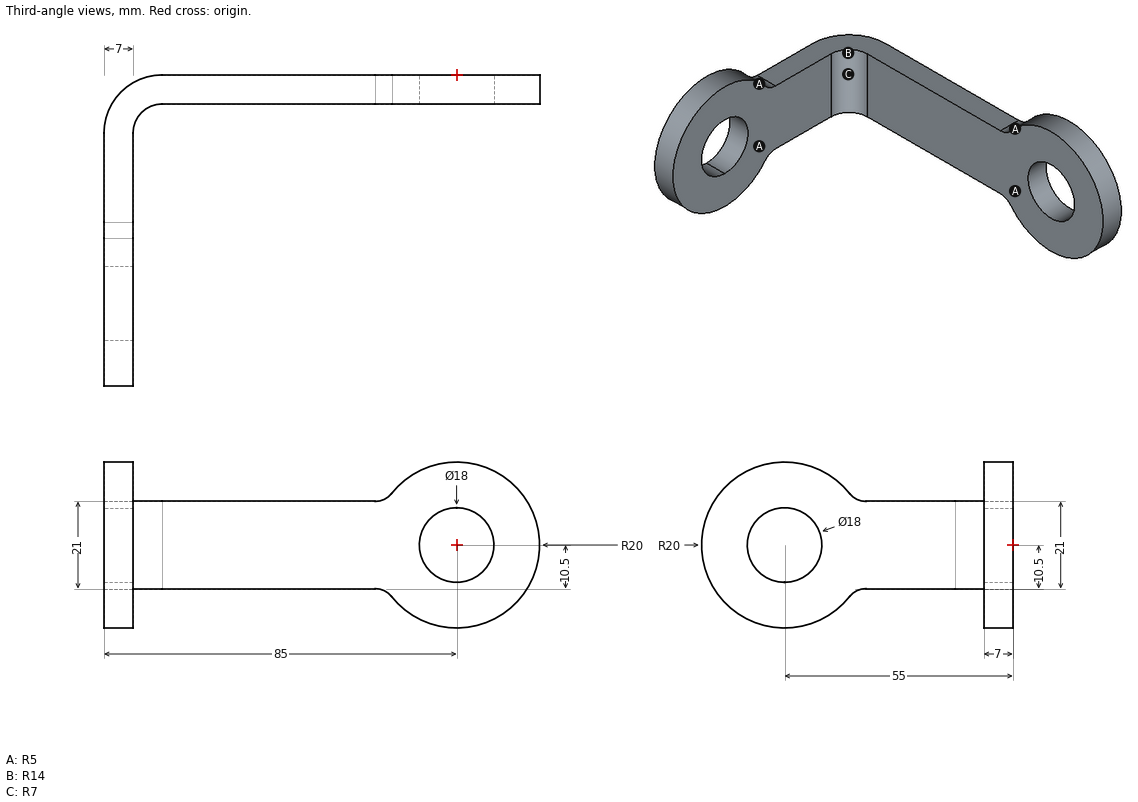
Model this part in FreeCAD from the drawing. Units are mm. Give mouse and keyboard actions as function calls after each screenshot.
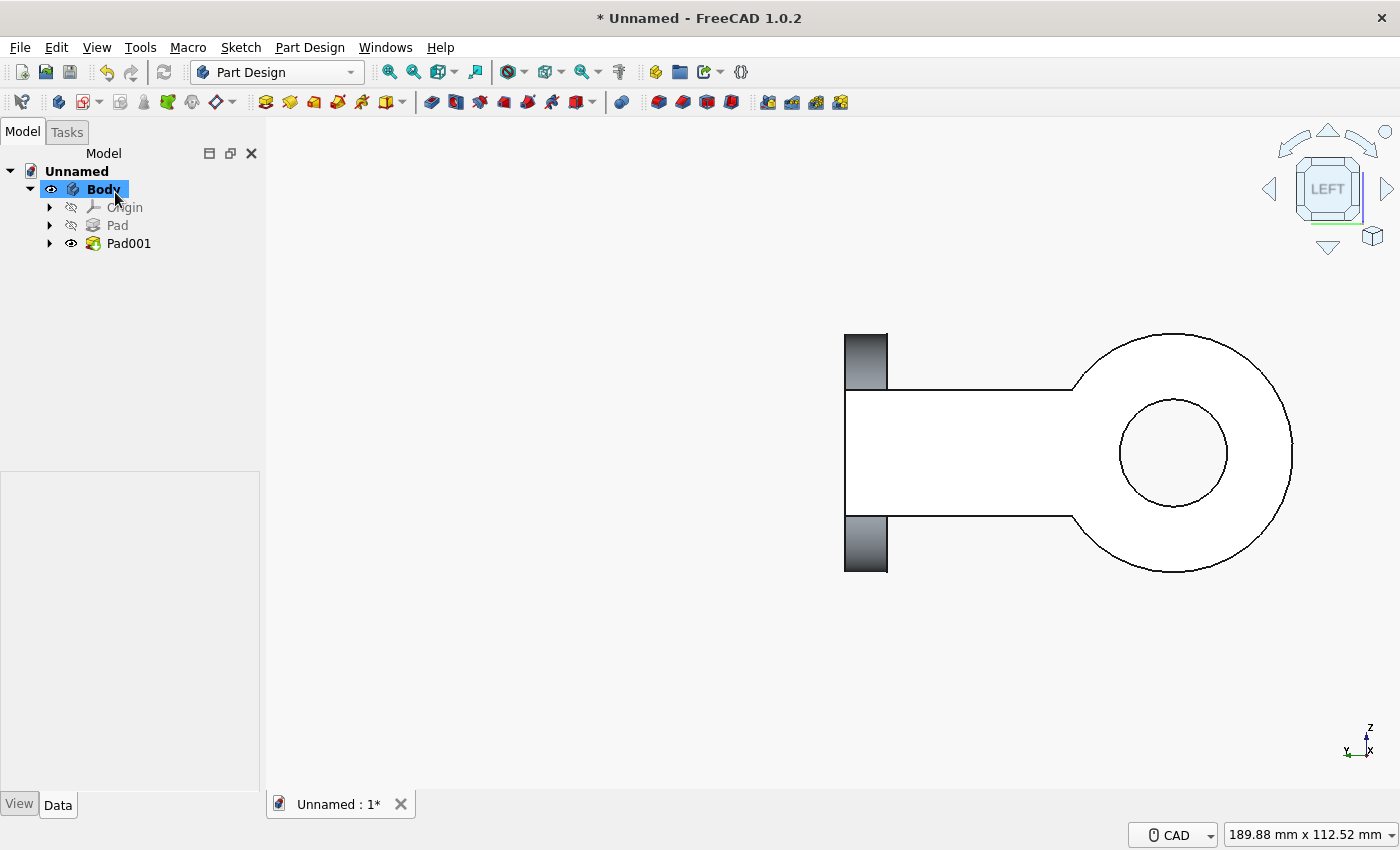
click(390, 72)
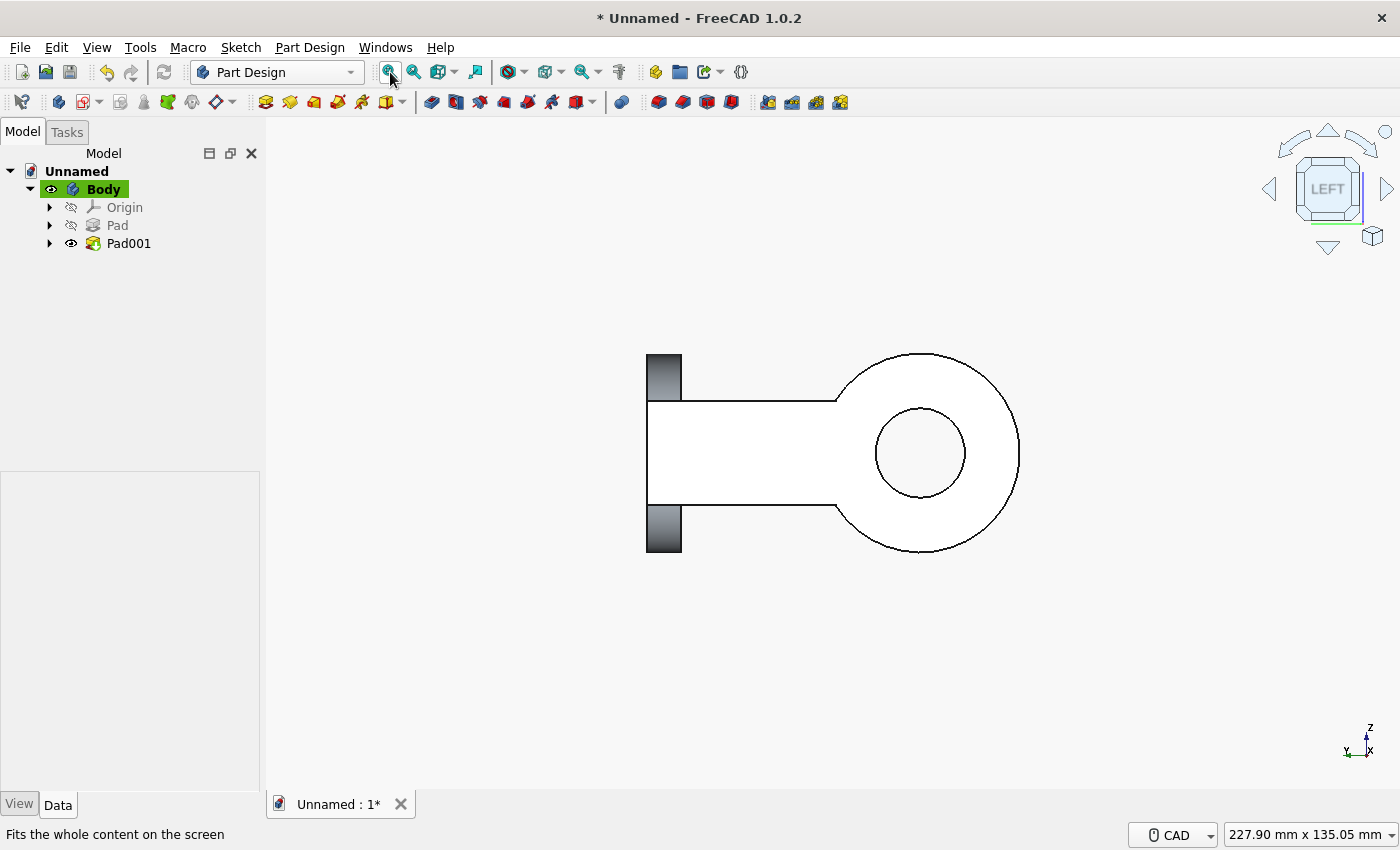
key(0)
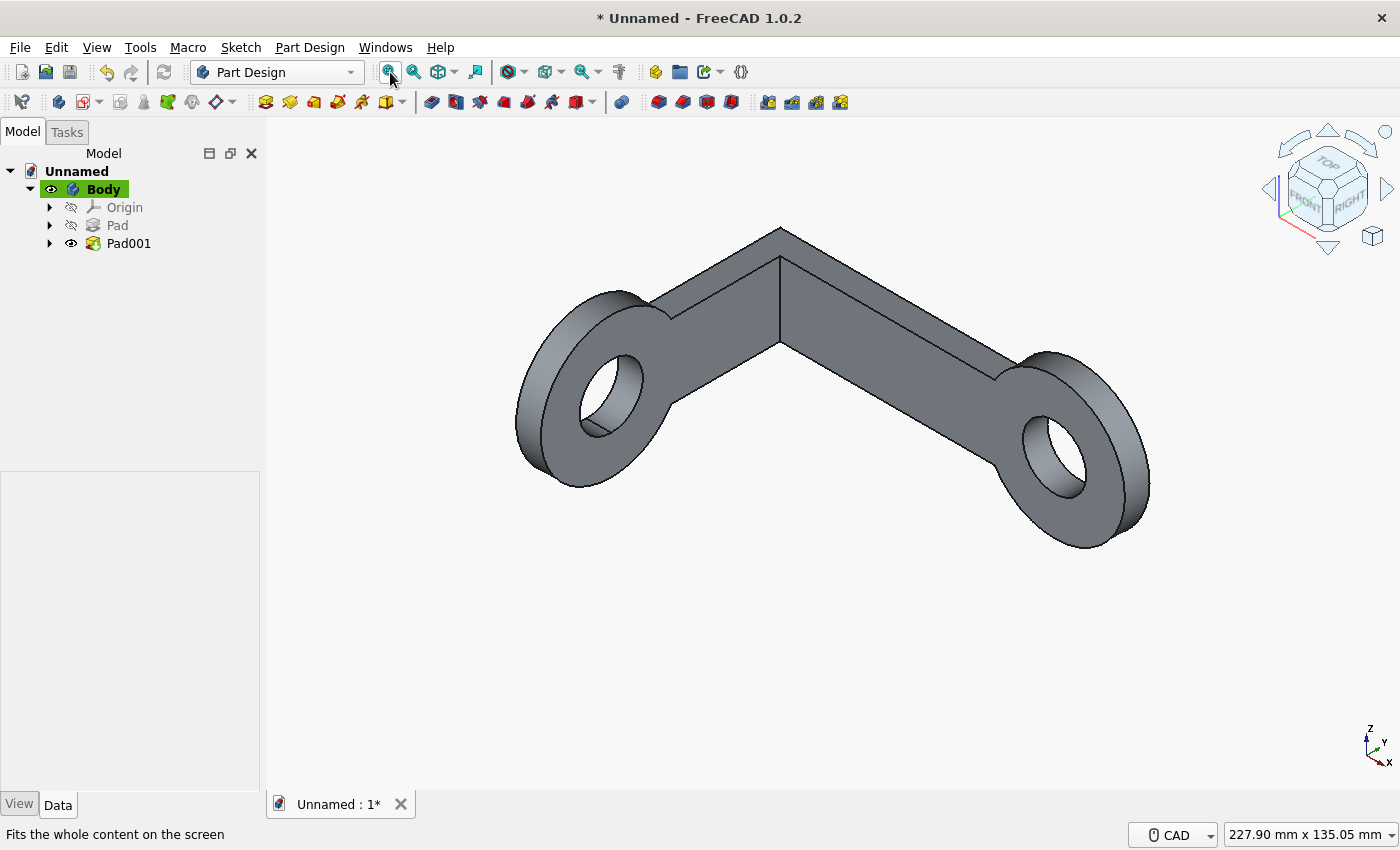
key(2)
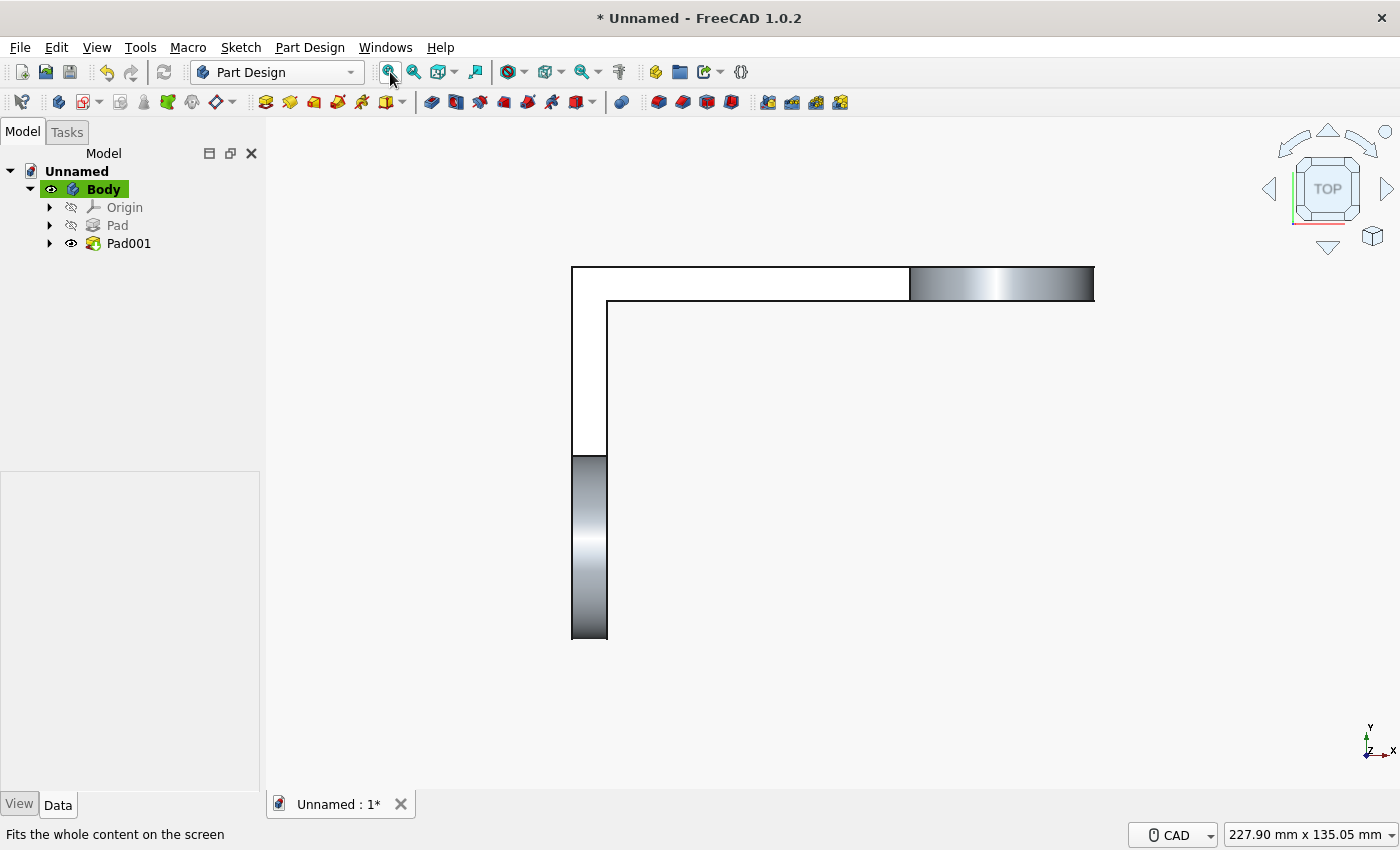
key(1)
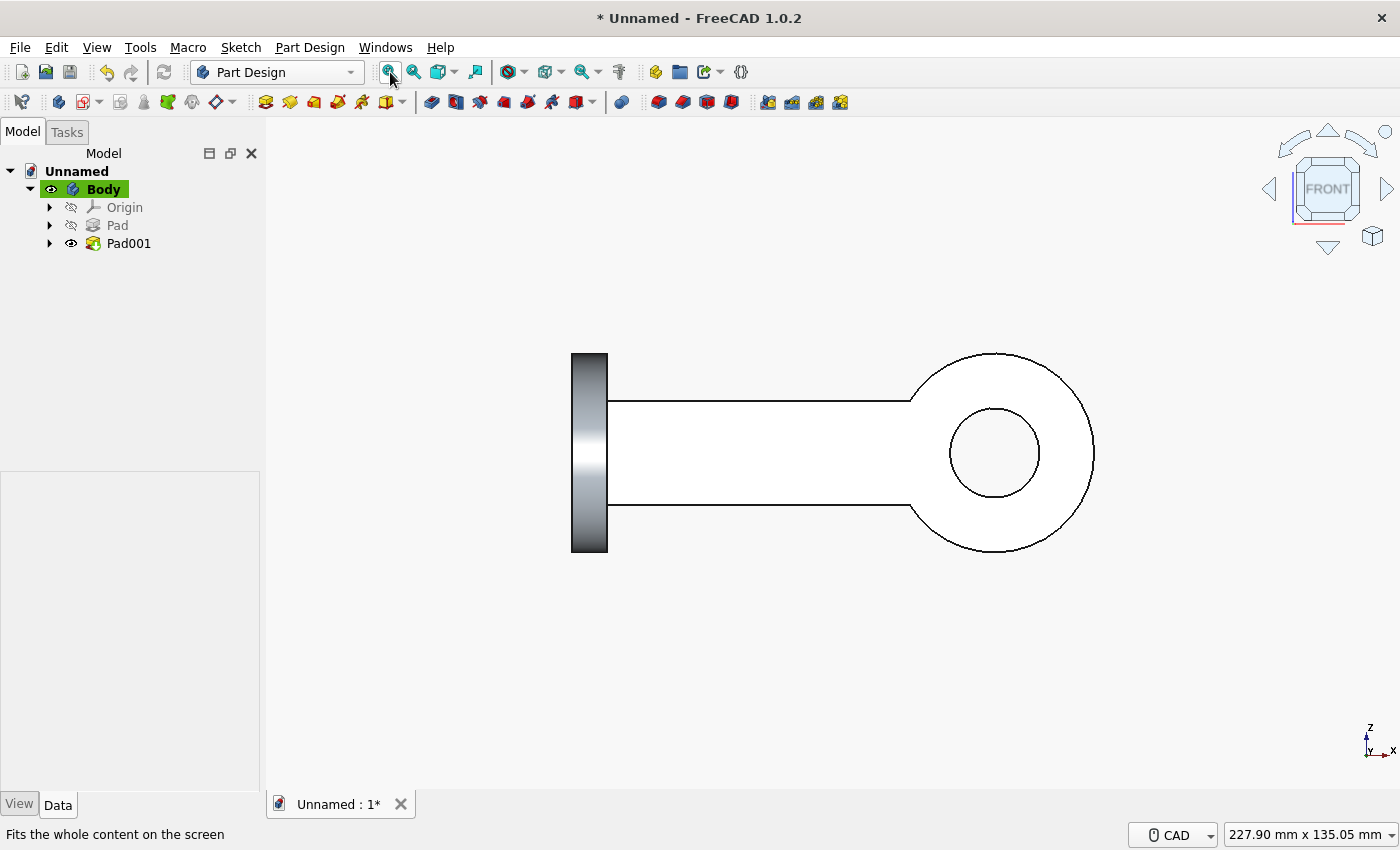
key(3)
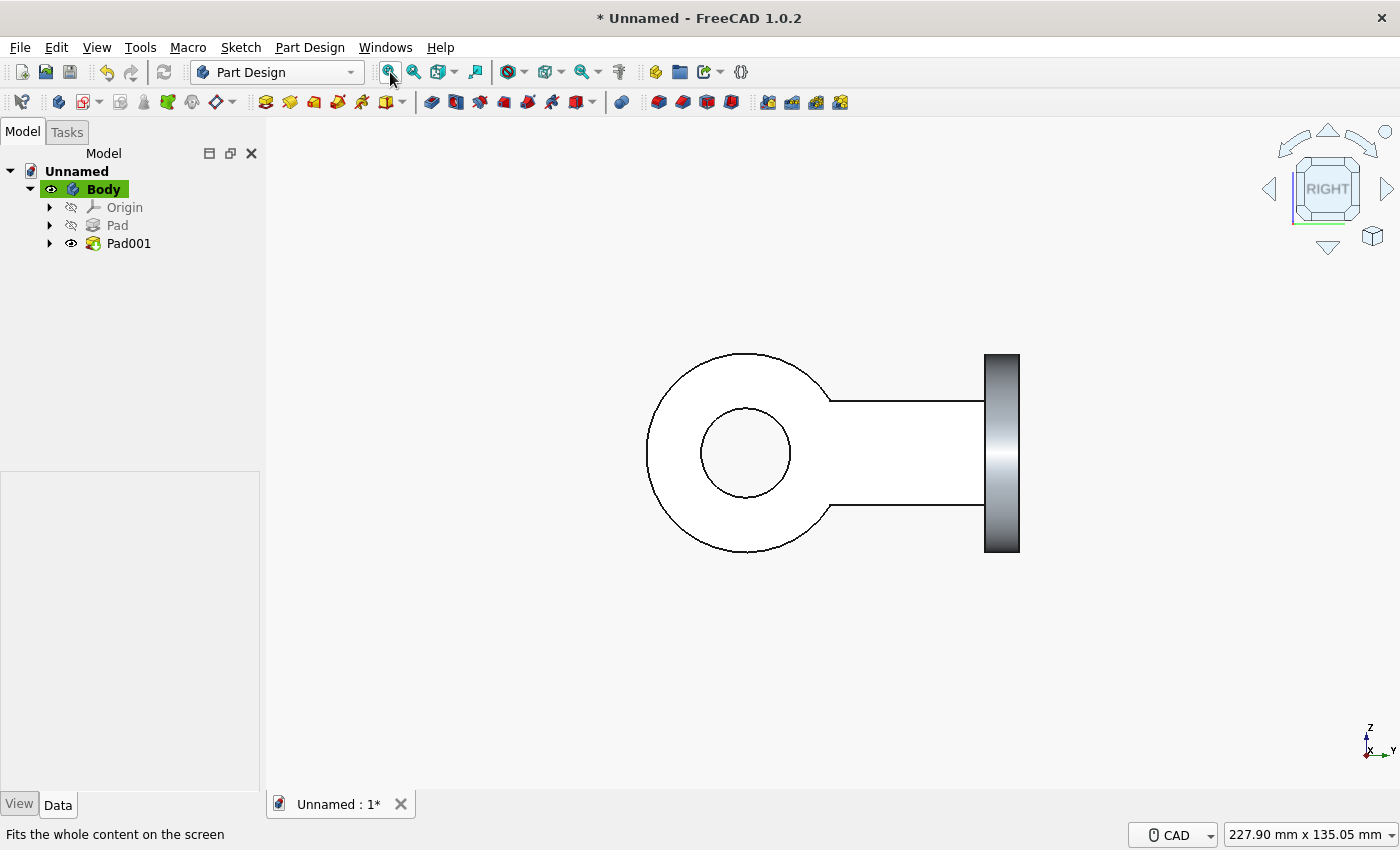
click(390, 72)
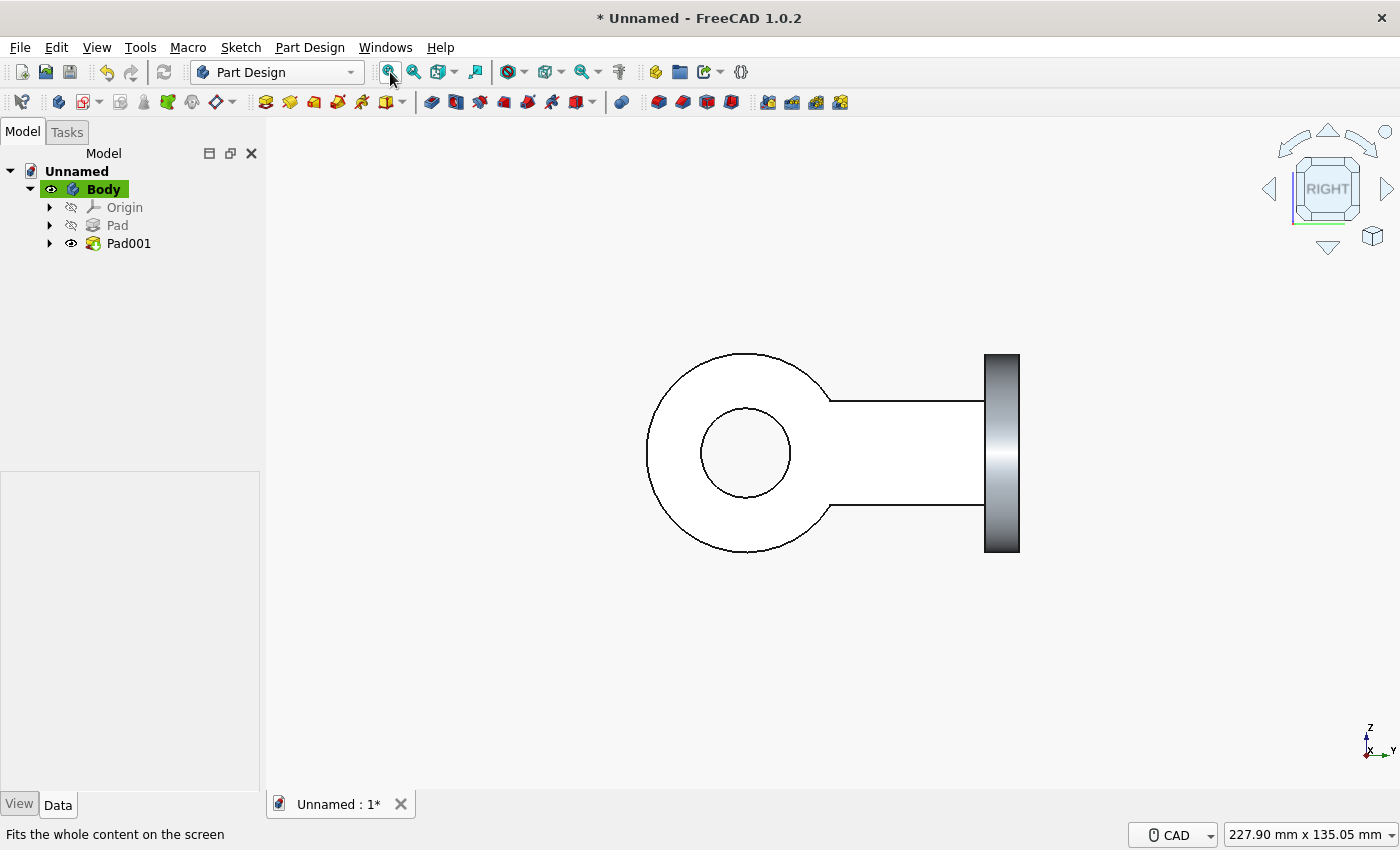
key(5)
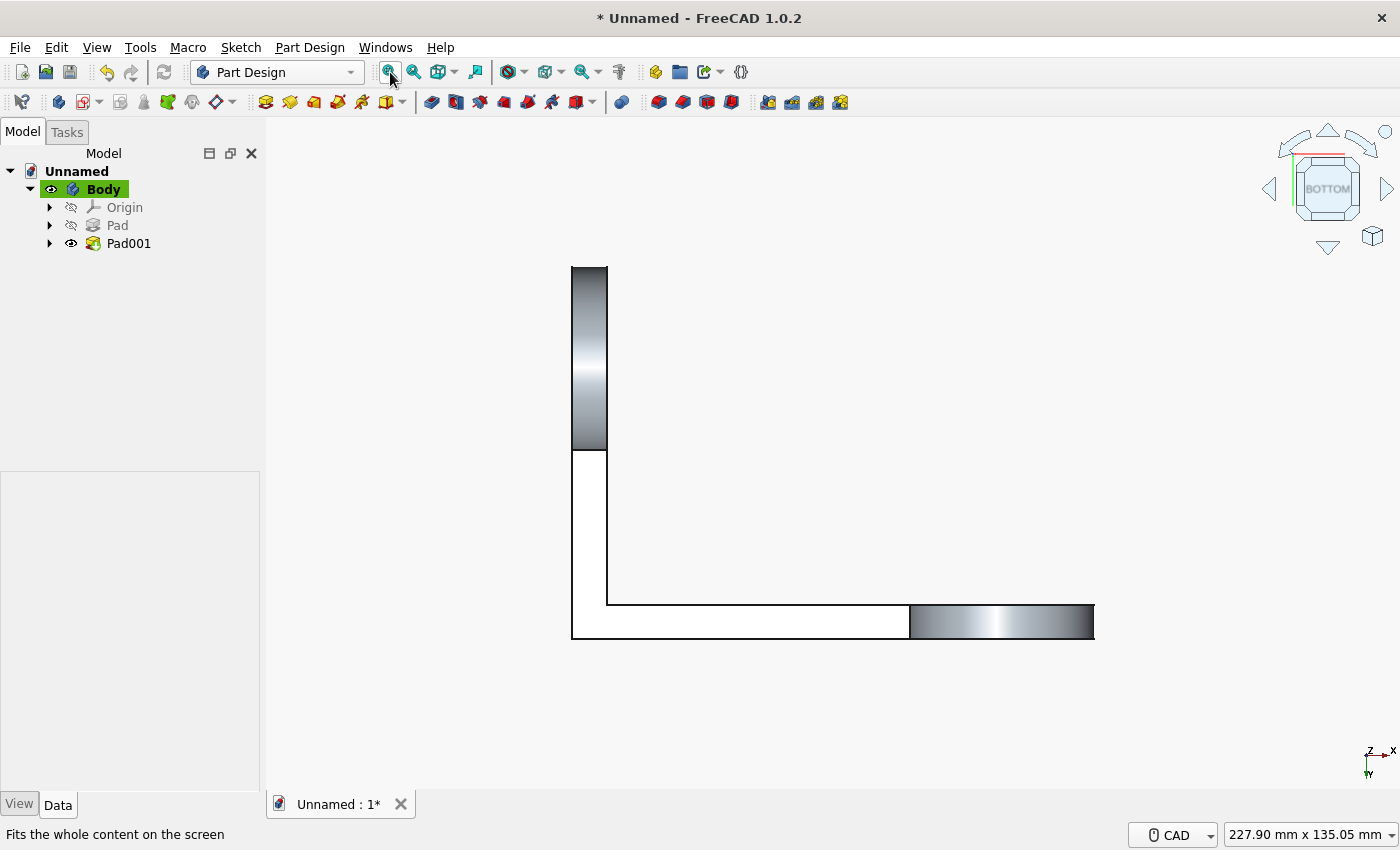
key(4)